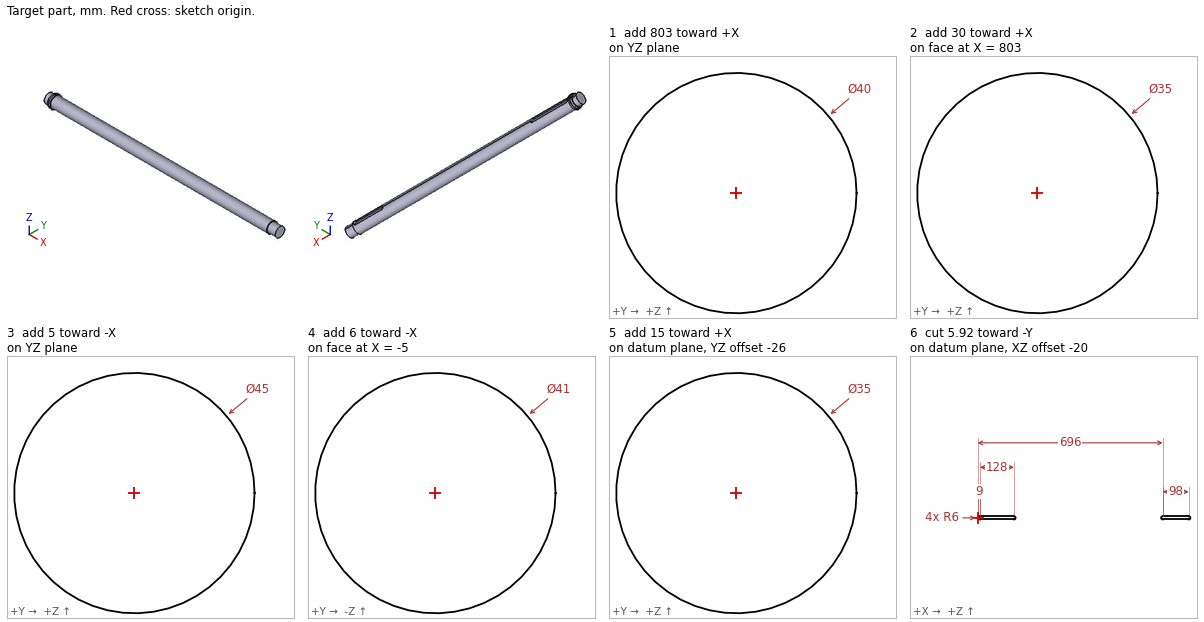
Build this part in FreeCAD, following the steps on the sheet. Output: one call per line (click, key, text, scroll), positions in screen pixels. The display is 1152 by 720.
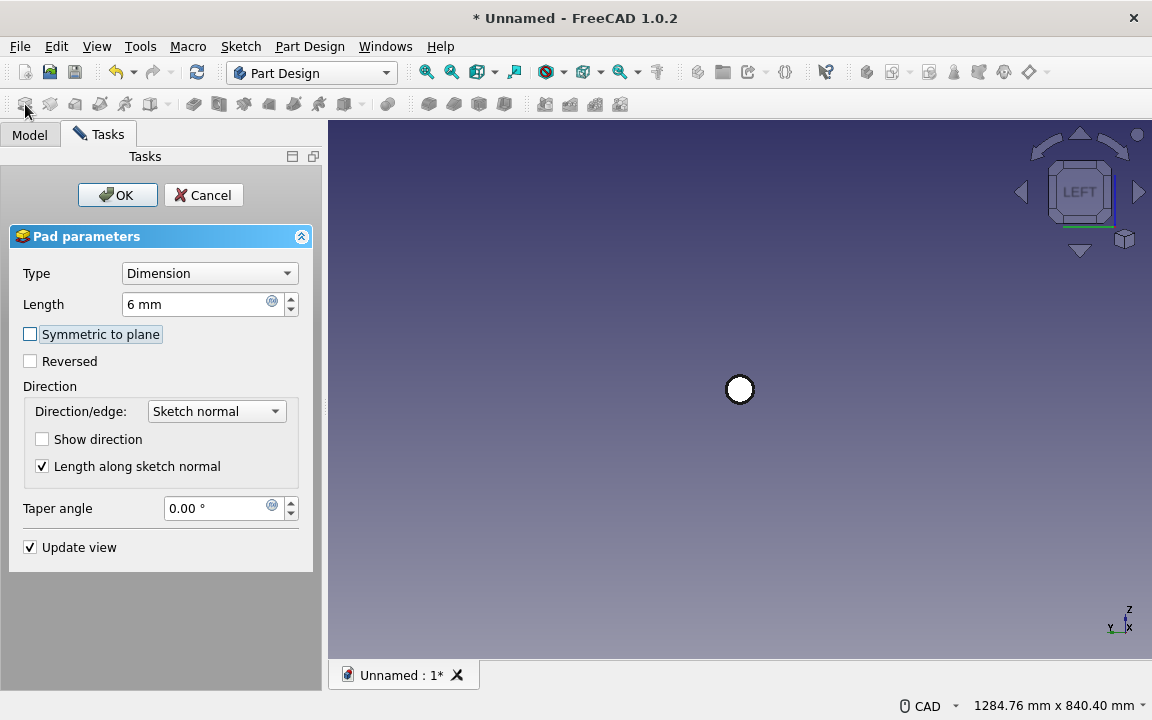
click(118, 195)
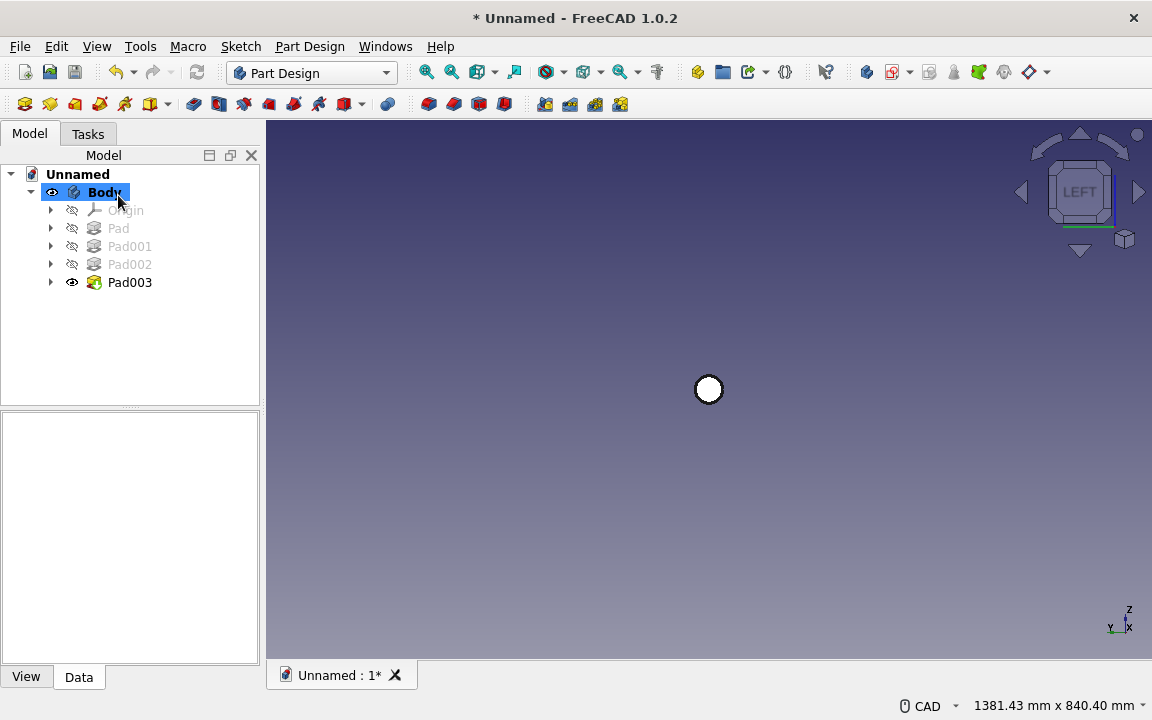
click(427, 72)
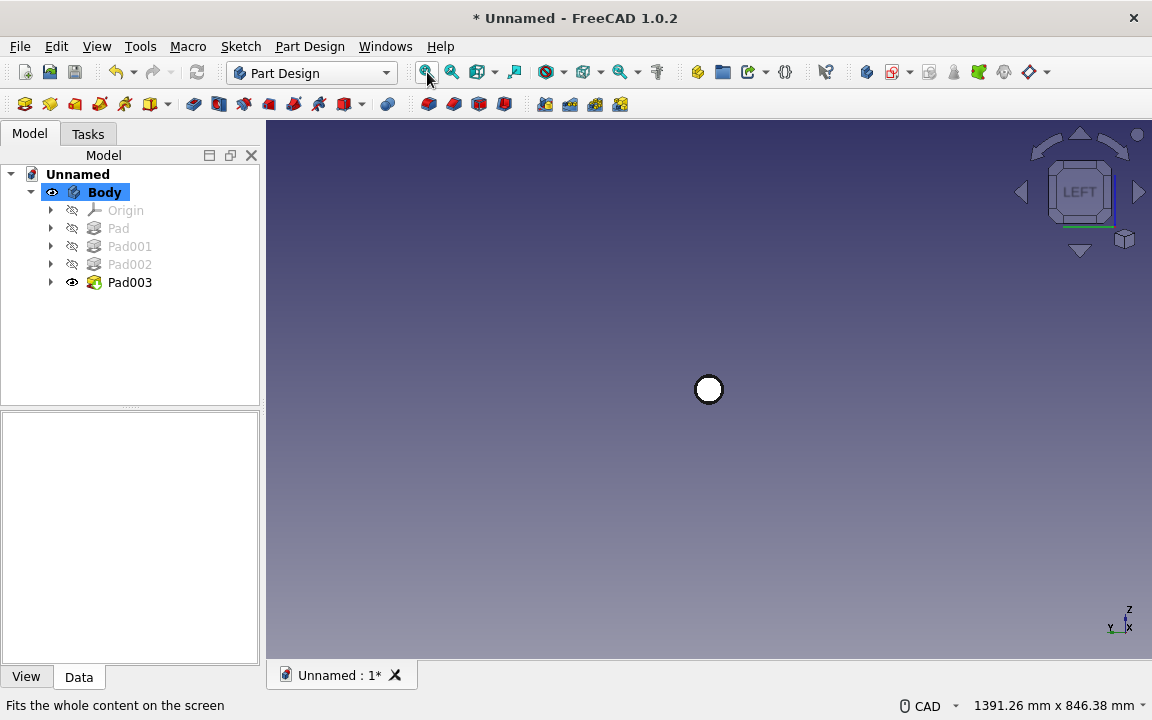
click(51, 210)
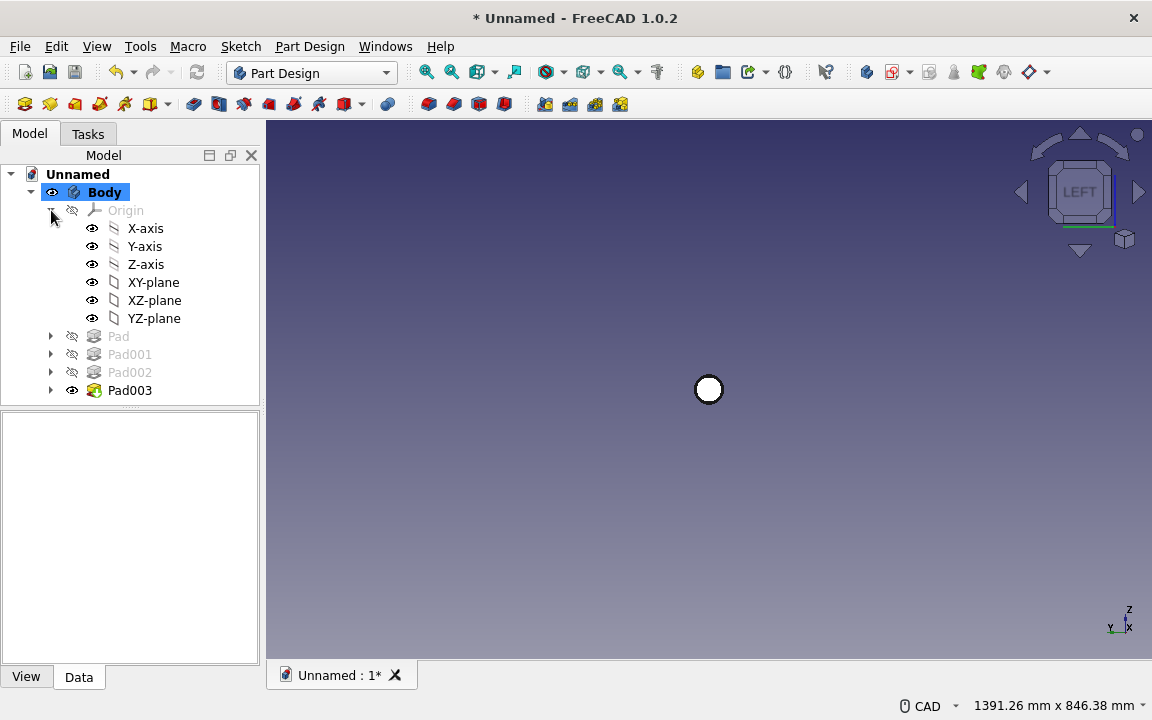
click(137, 318)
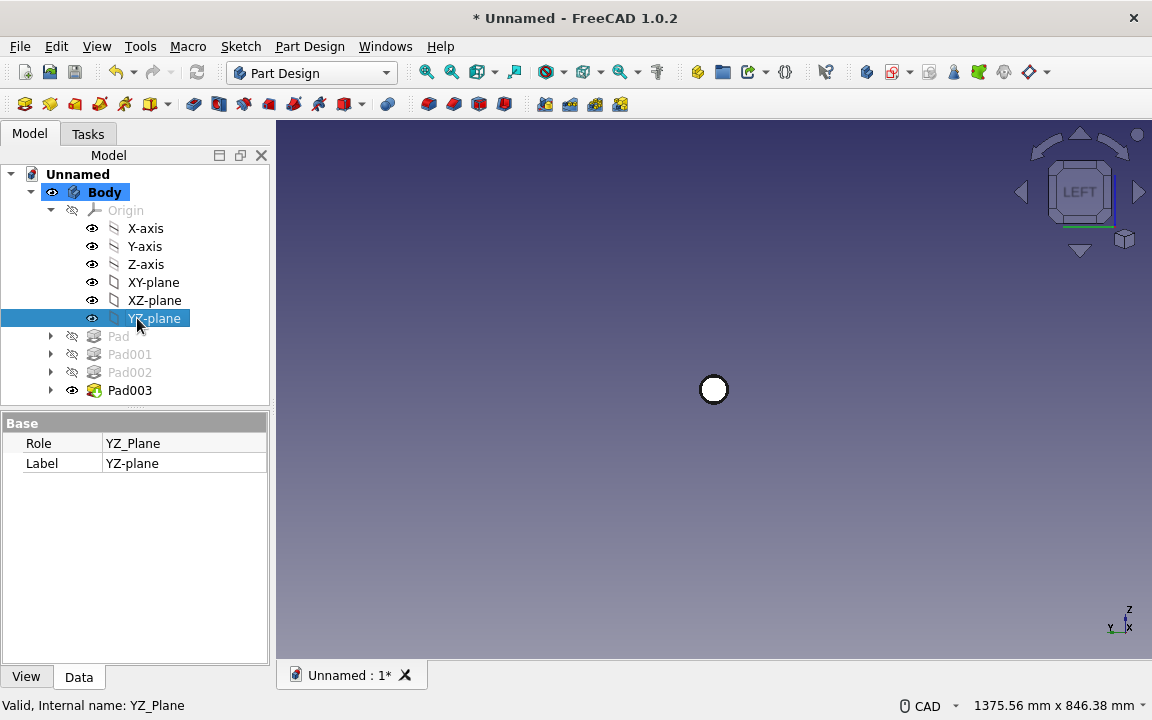
click(1028, 72)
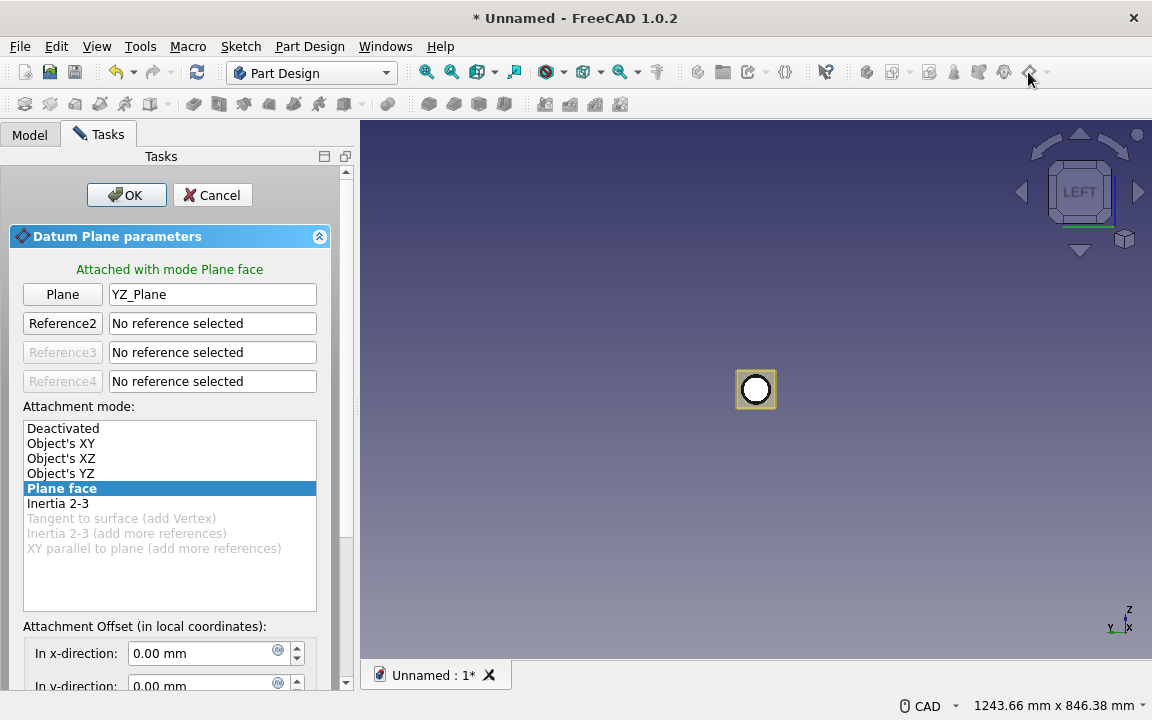
scroll(346, 428, down, 2)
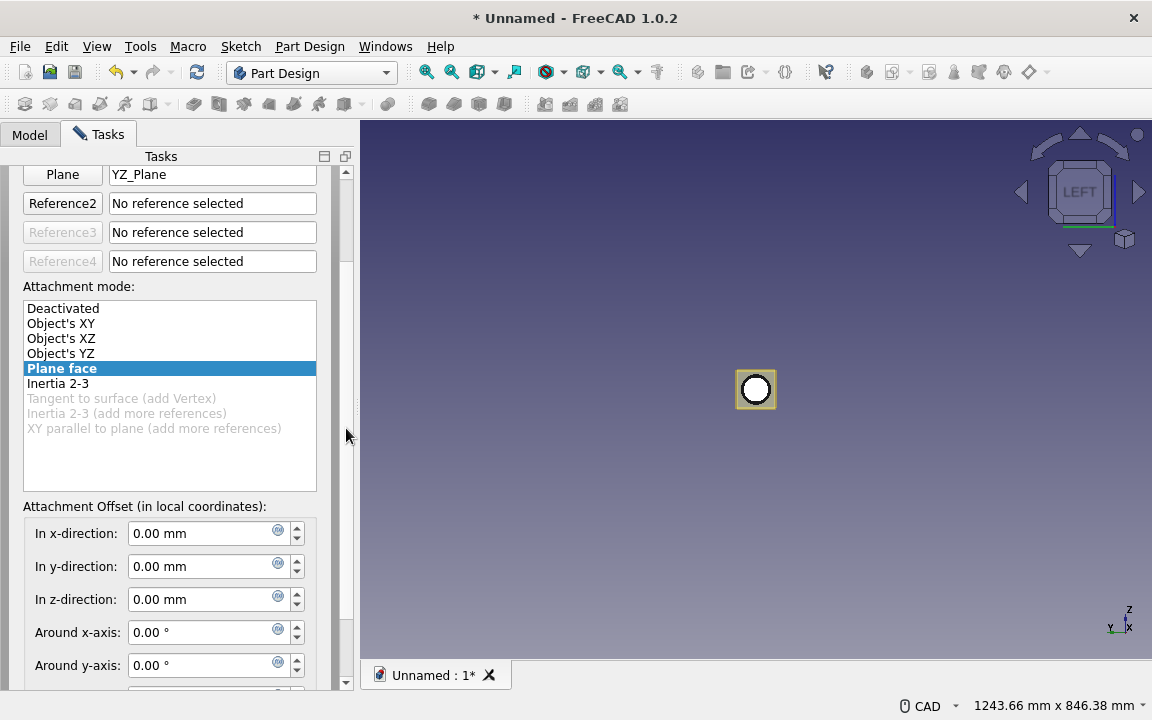
triple_click(210, 600)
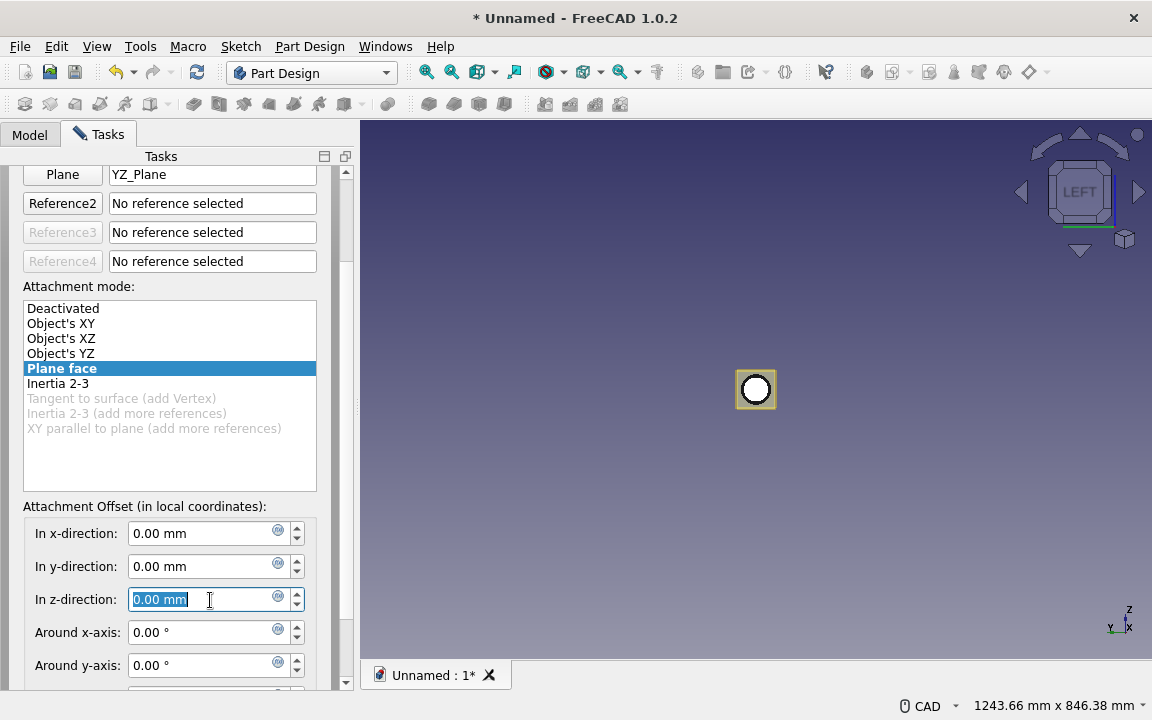
text(-26)
key(Tab)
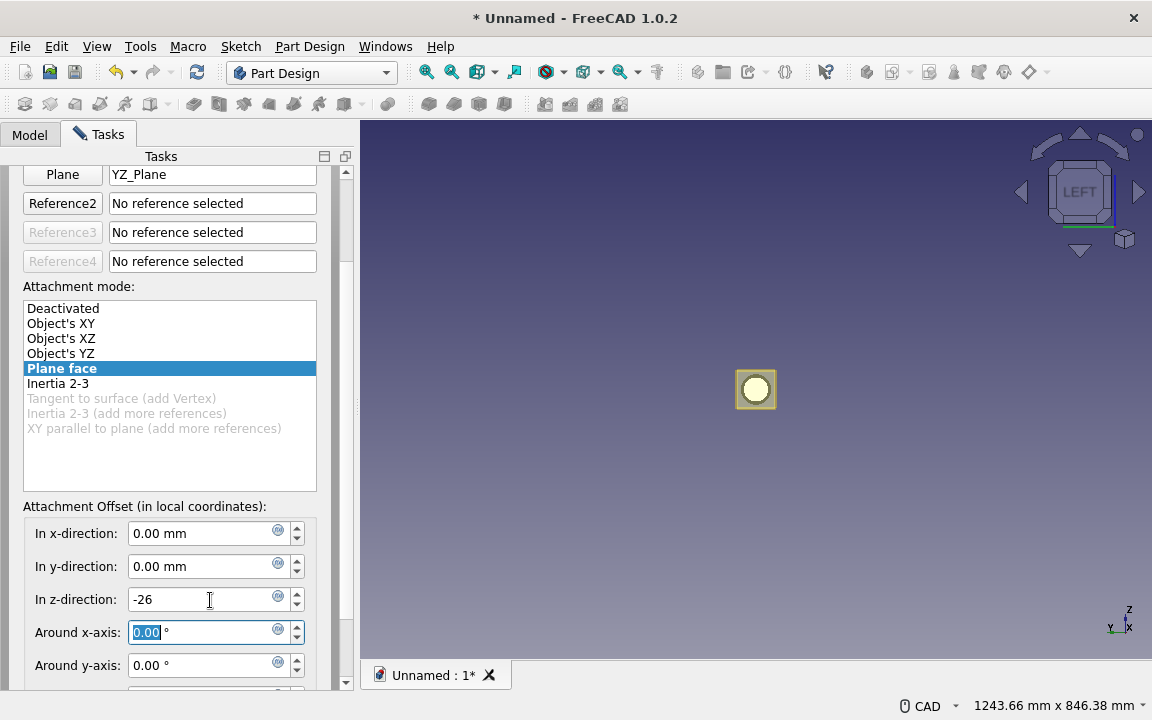
scroll(346, 428, up, 3)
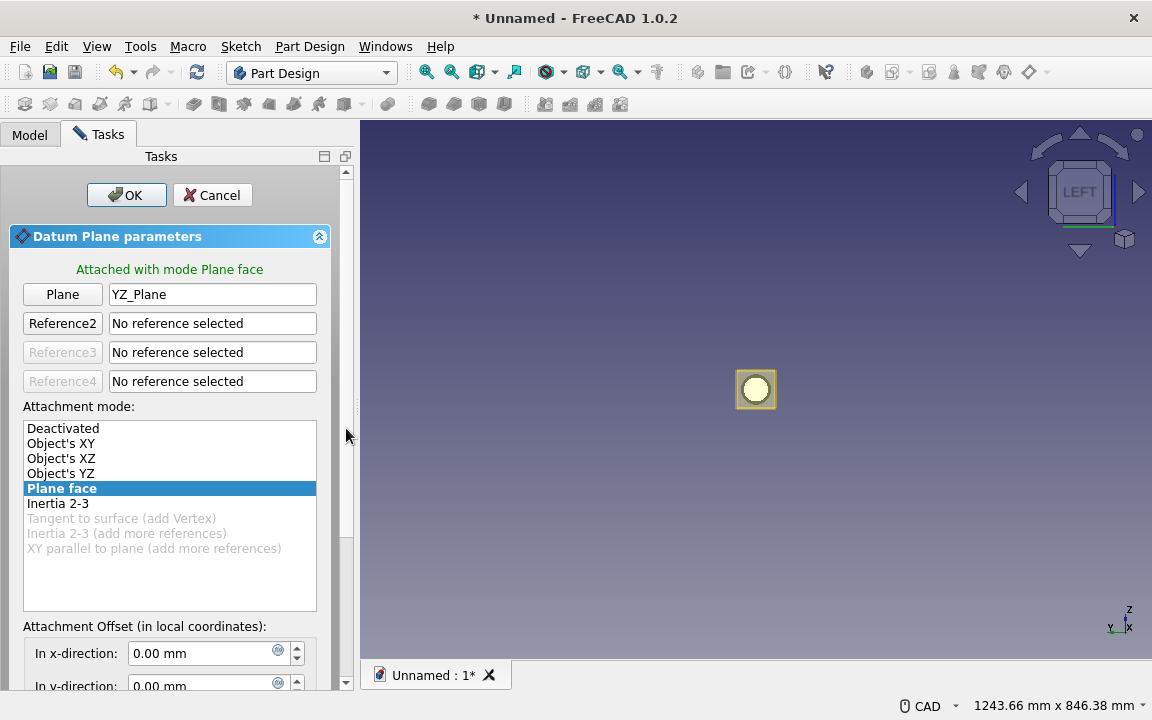
click(127, 195)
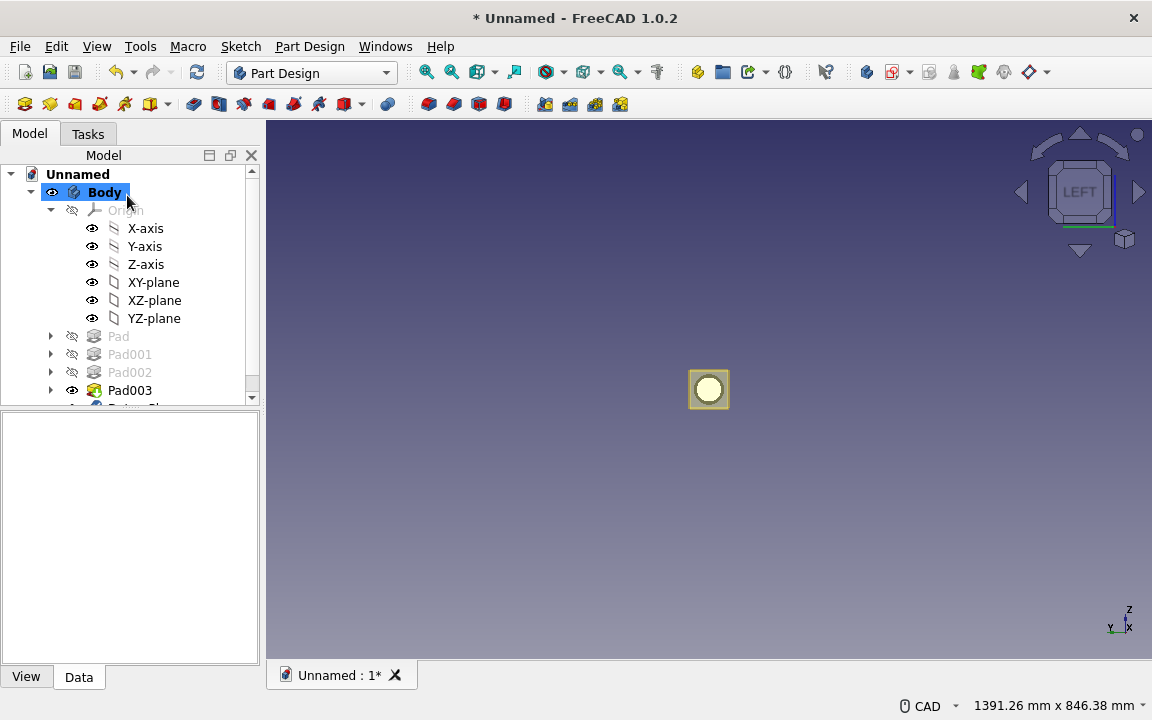
scroll(101, 278, down, 3)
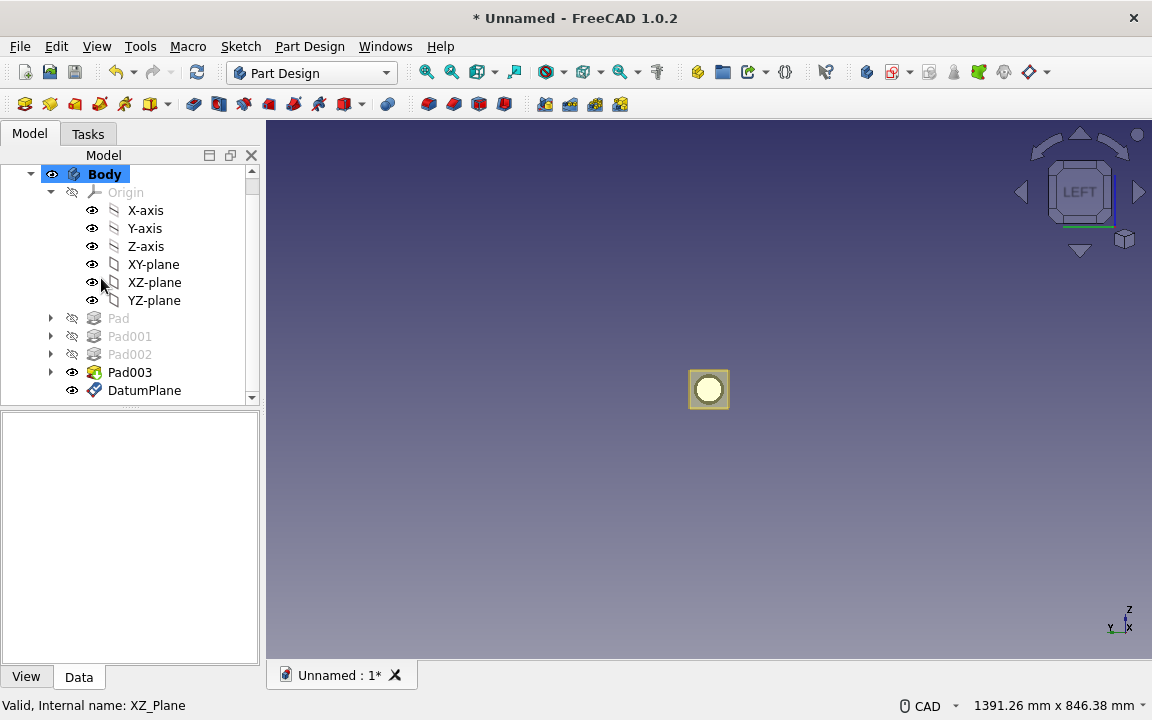
click(117, 390)